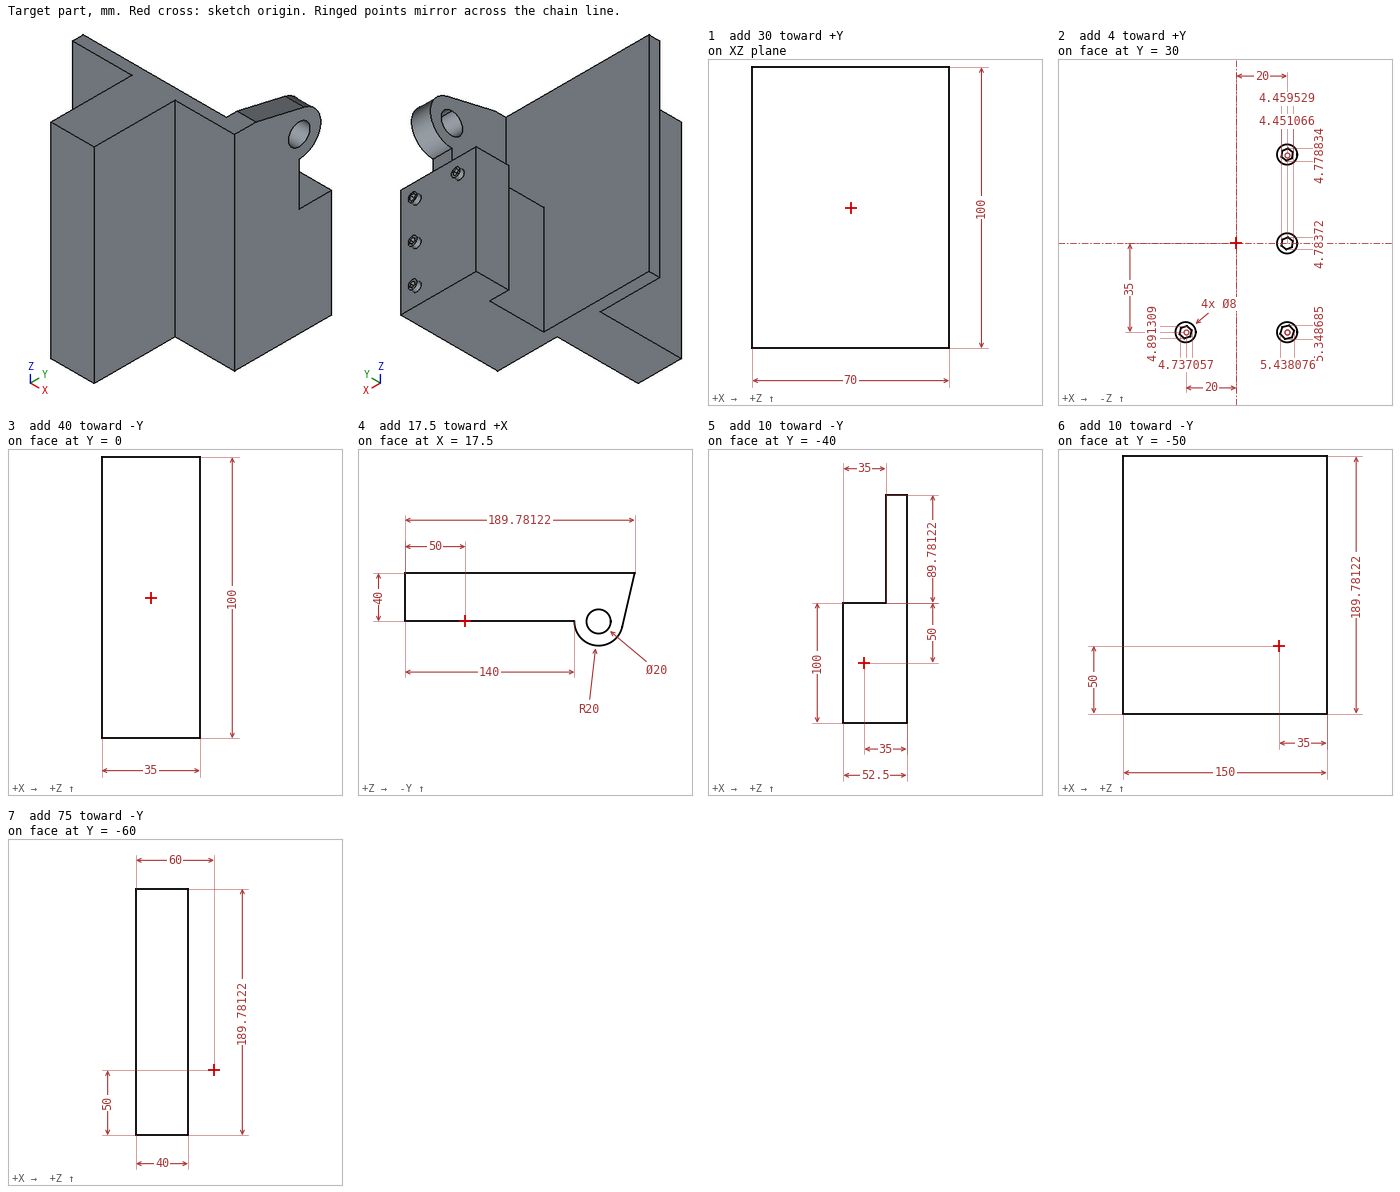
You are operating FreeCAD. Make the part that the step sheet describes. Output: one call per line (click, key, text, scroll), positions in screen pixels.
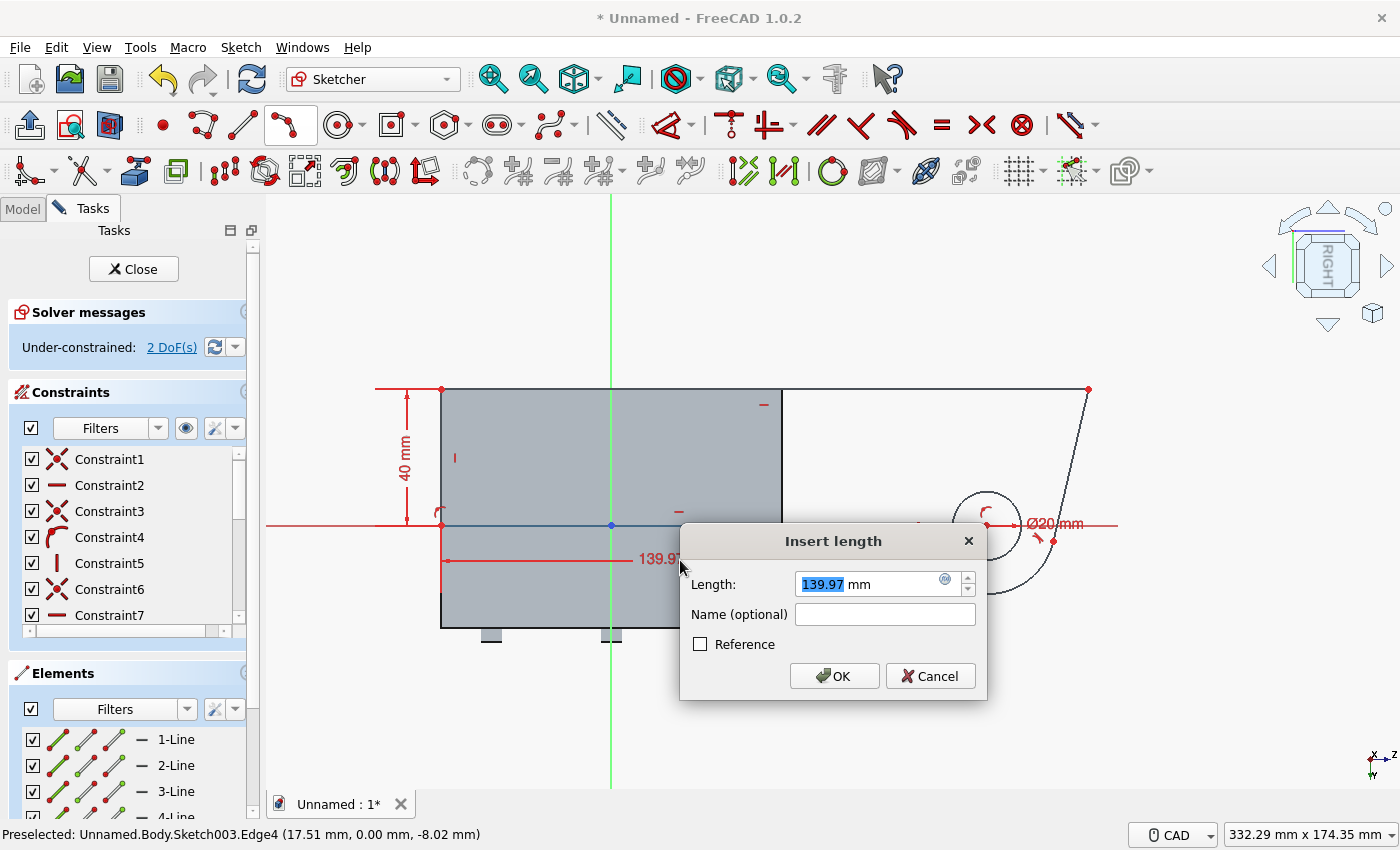
text(140)
key(Return)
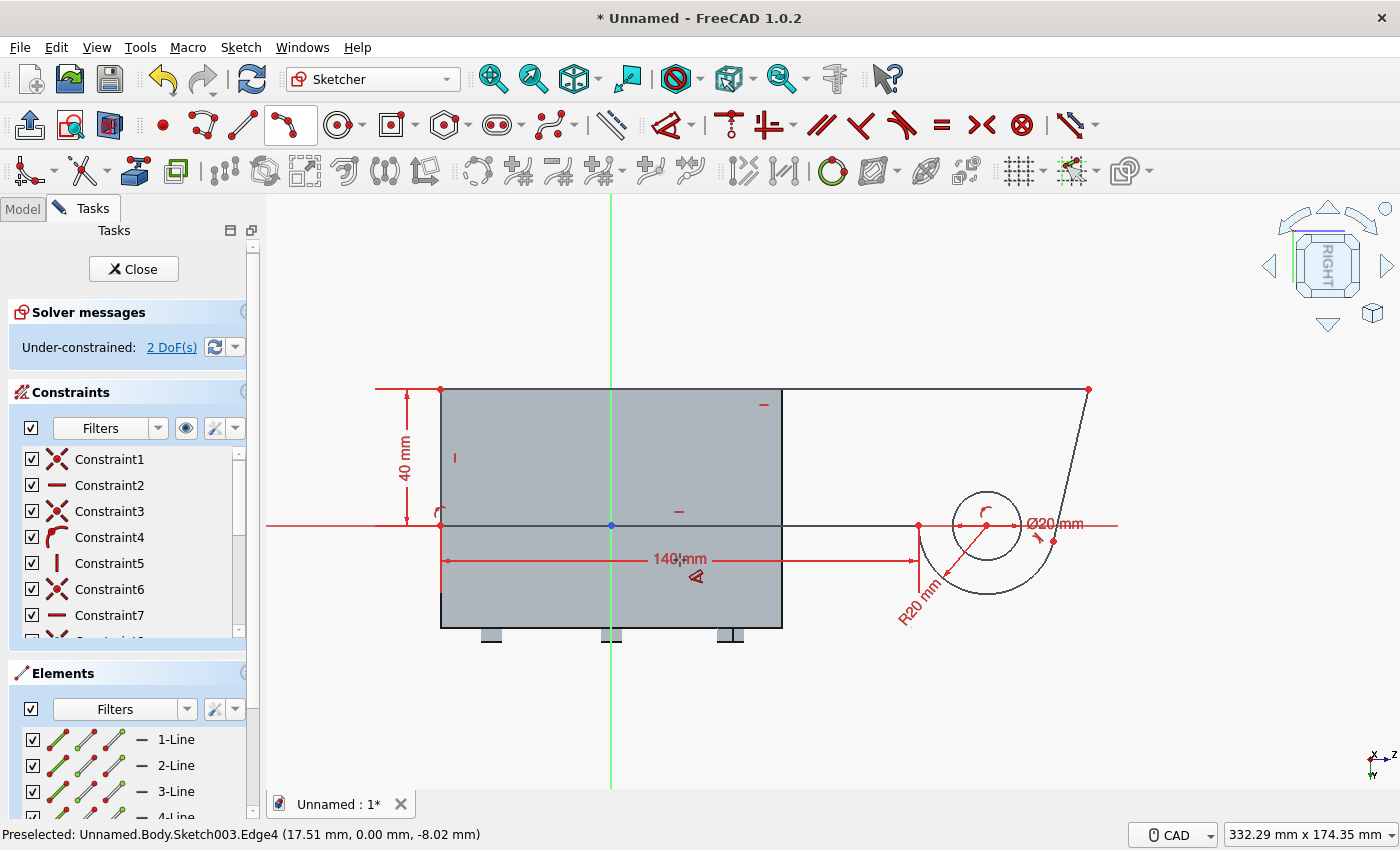
click(441, 389)
click(526, 355)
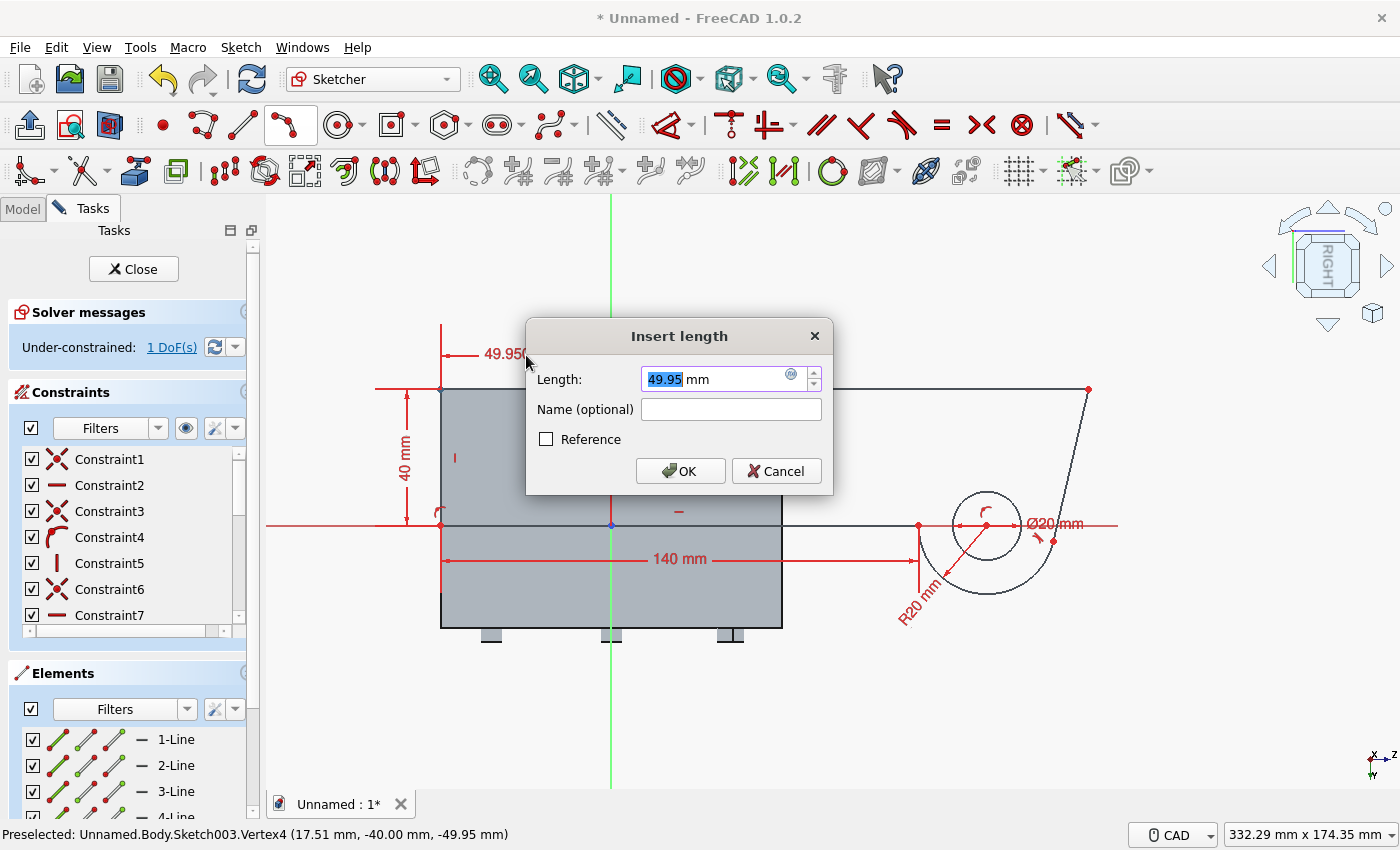
text(50)
key(Return)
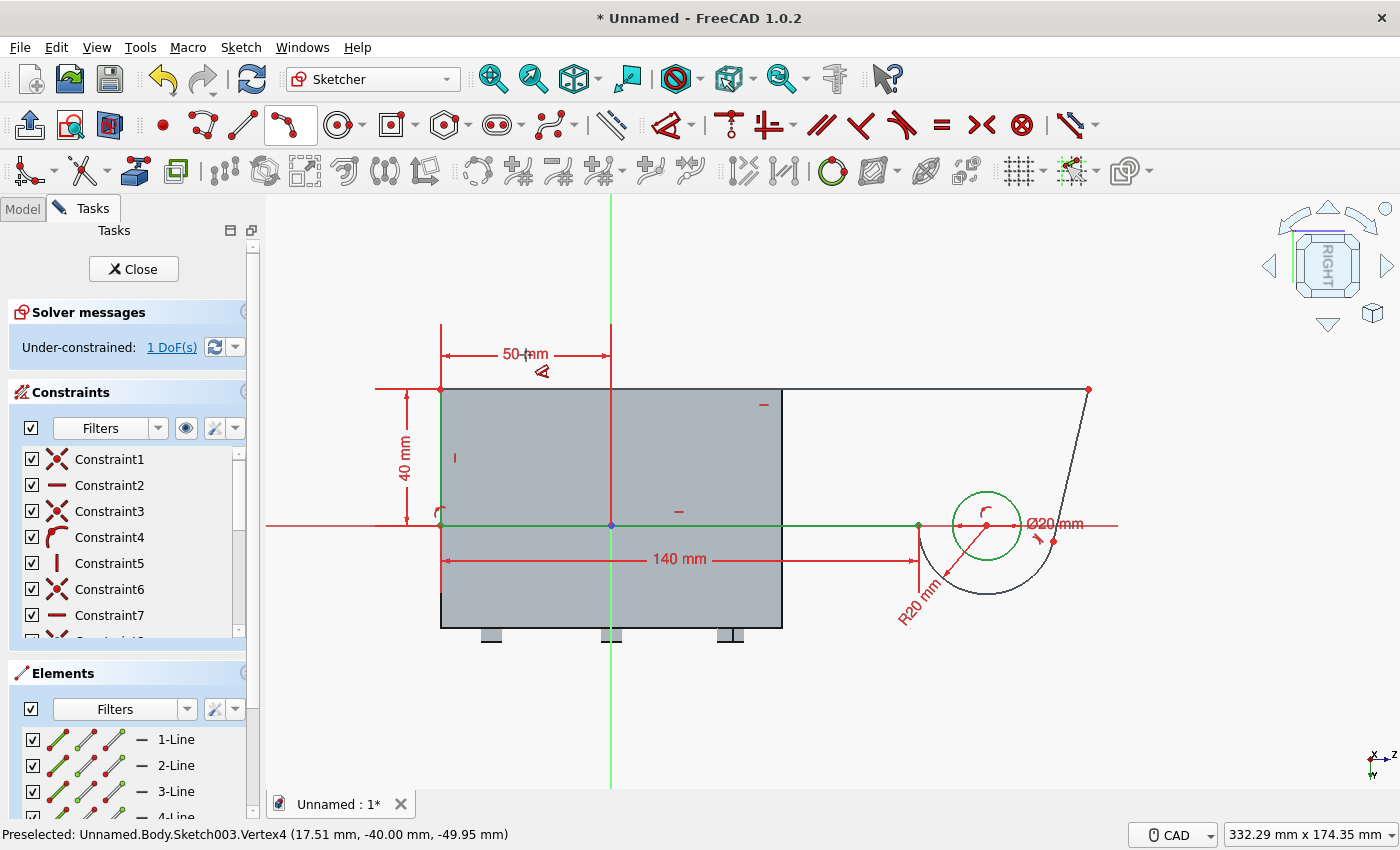
click(894, 389)
click(765, 355)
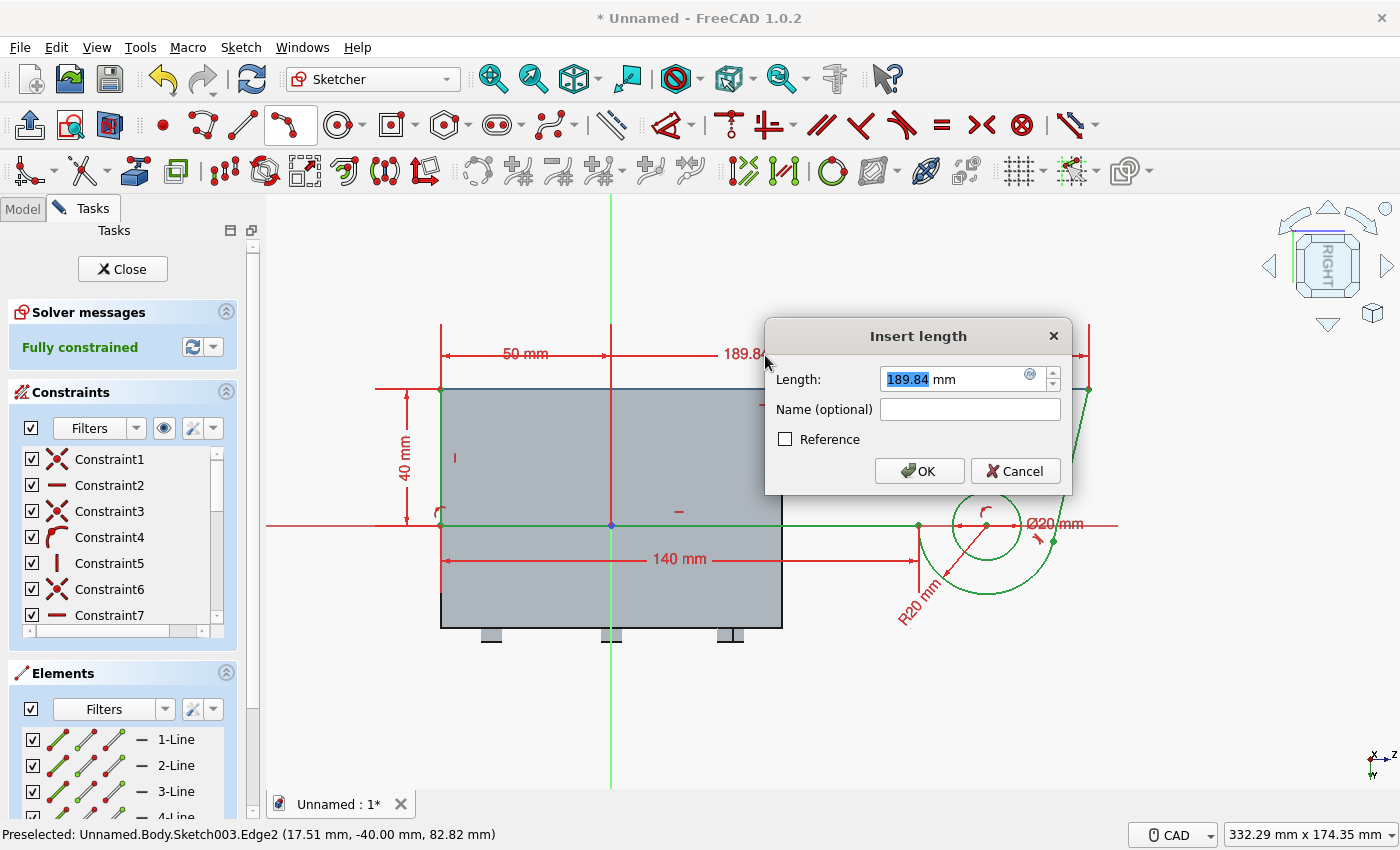
text(189.78122)
key(Return)
key(Escape)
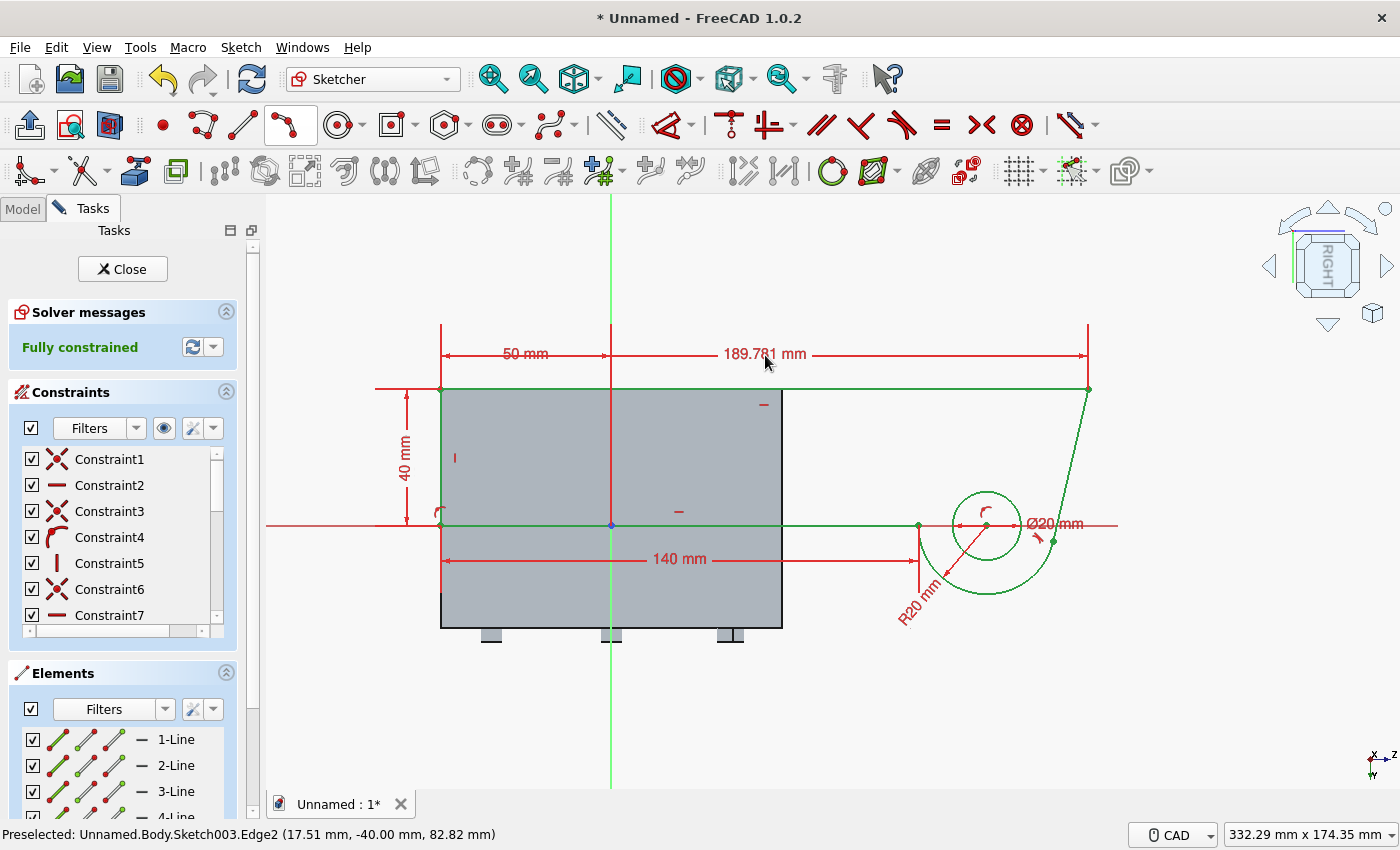
click(123, 269)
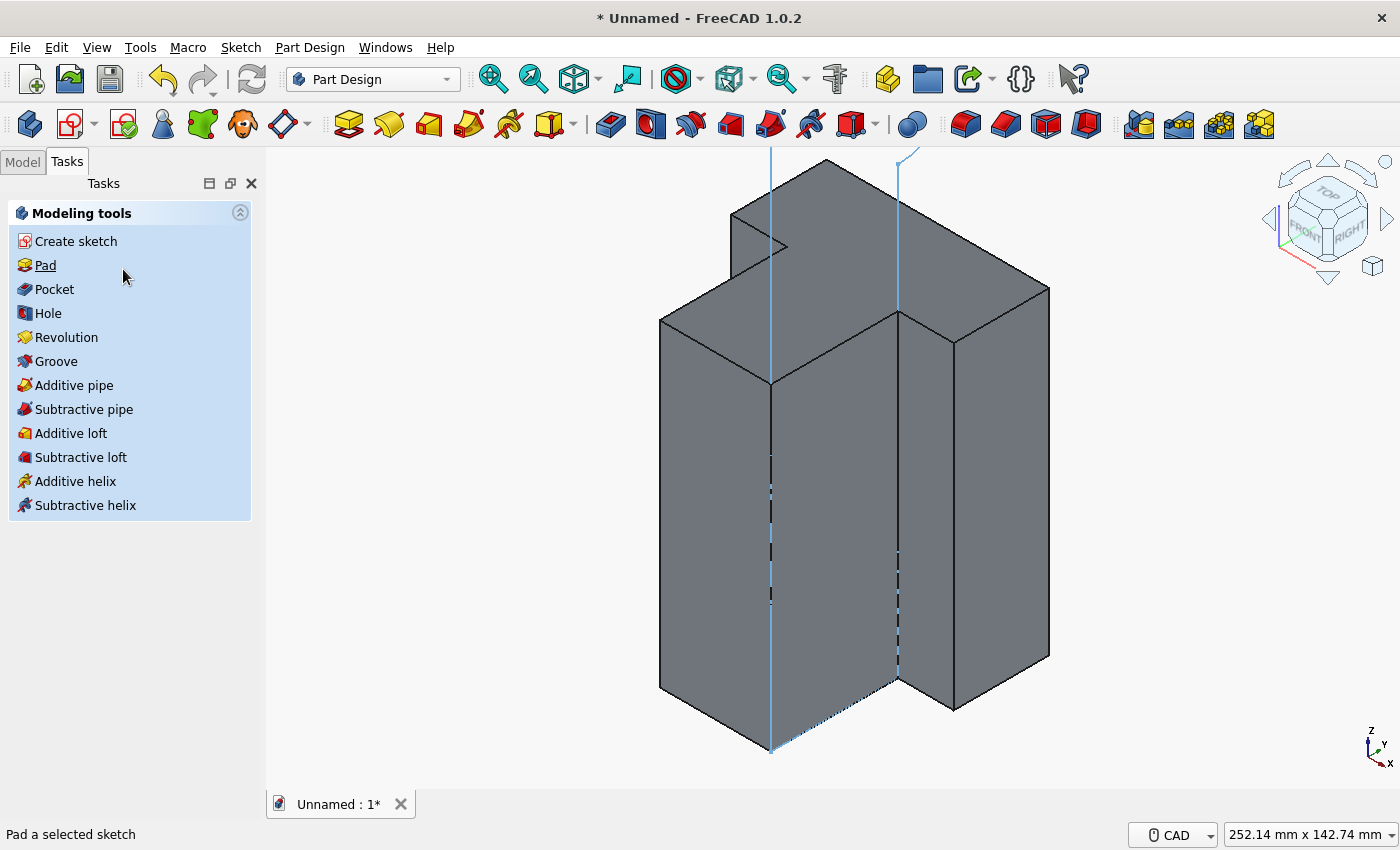
click(350, 124)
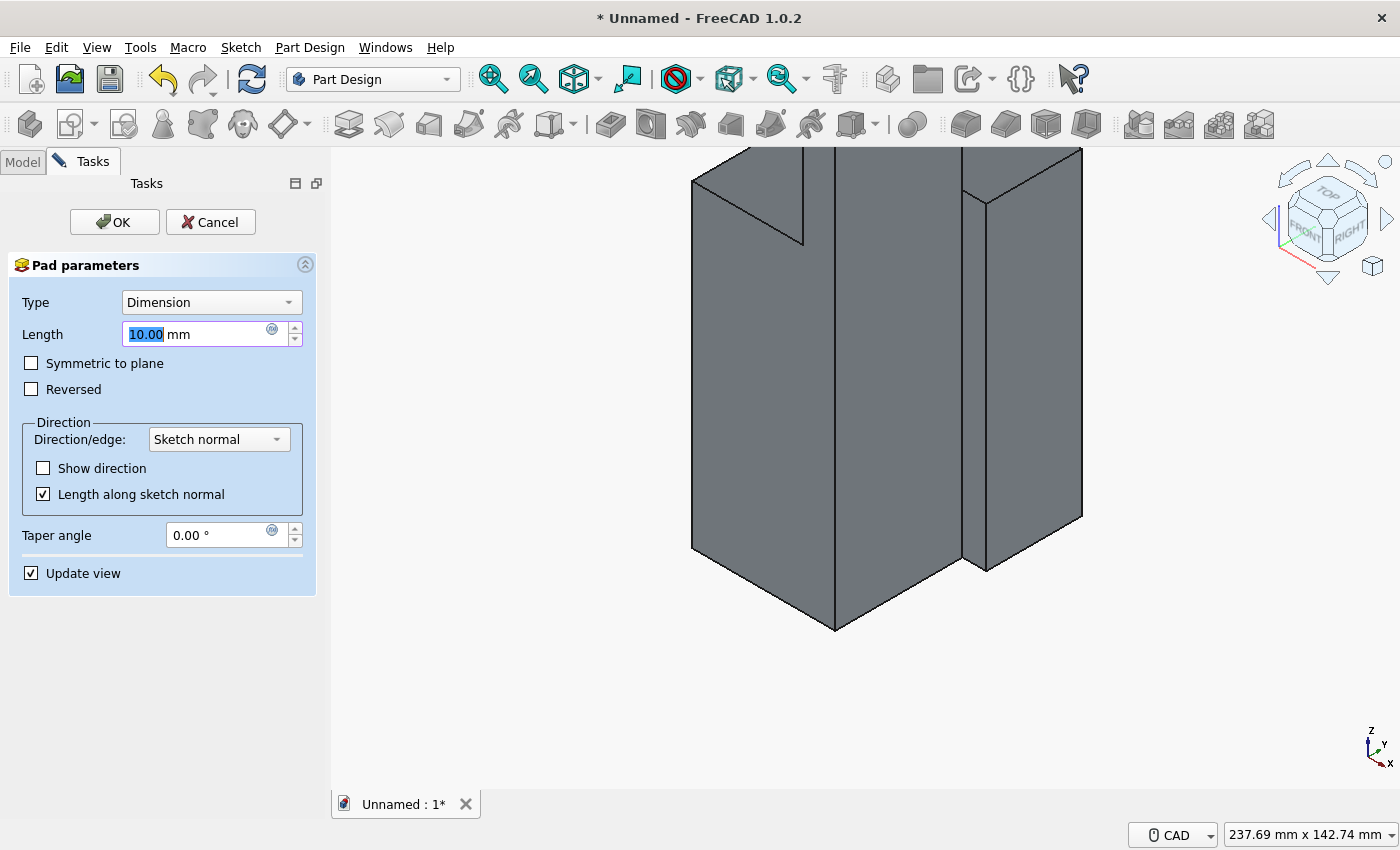
text(17.5)
key(Tab)